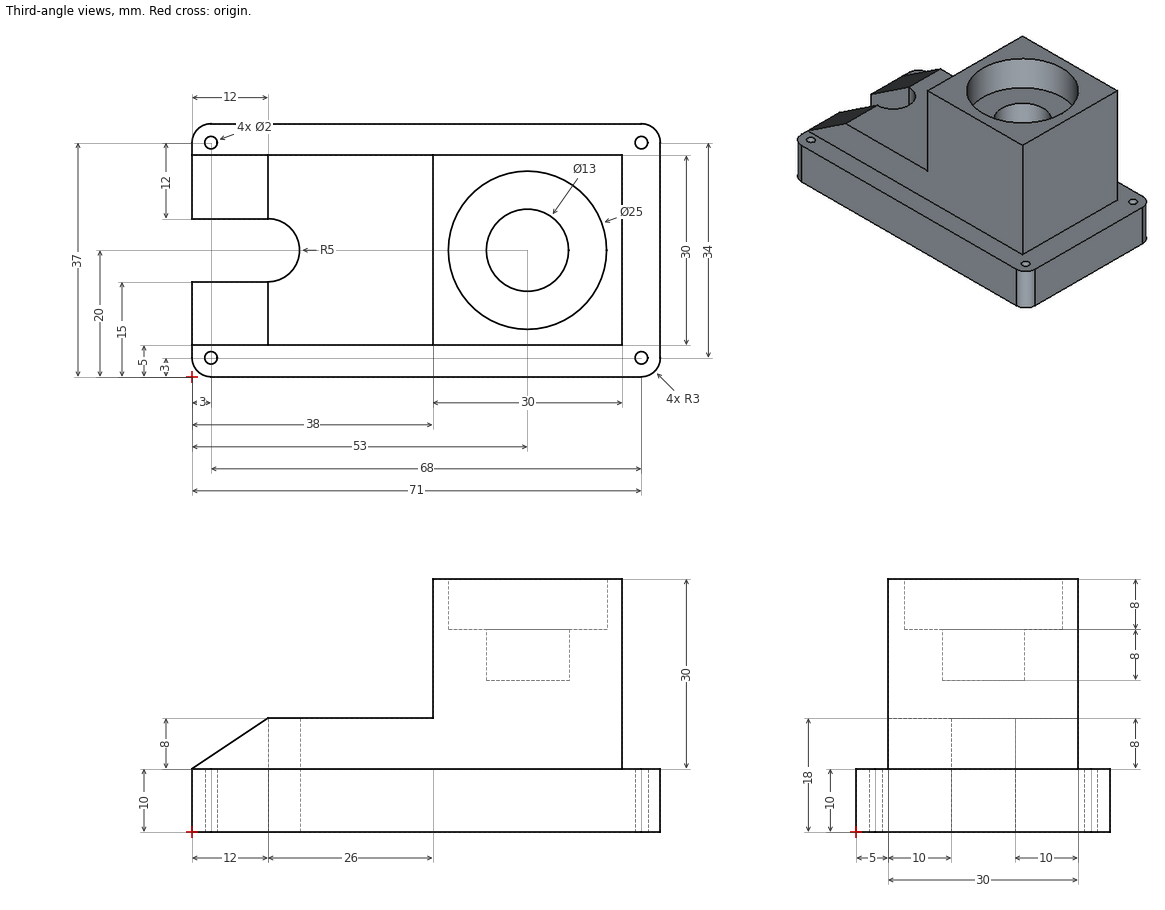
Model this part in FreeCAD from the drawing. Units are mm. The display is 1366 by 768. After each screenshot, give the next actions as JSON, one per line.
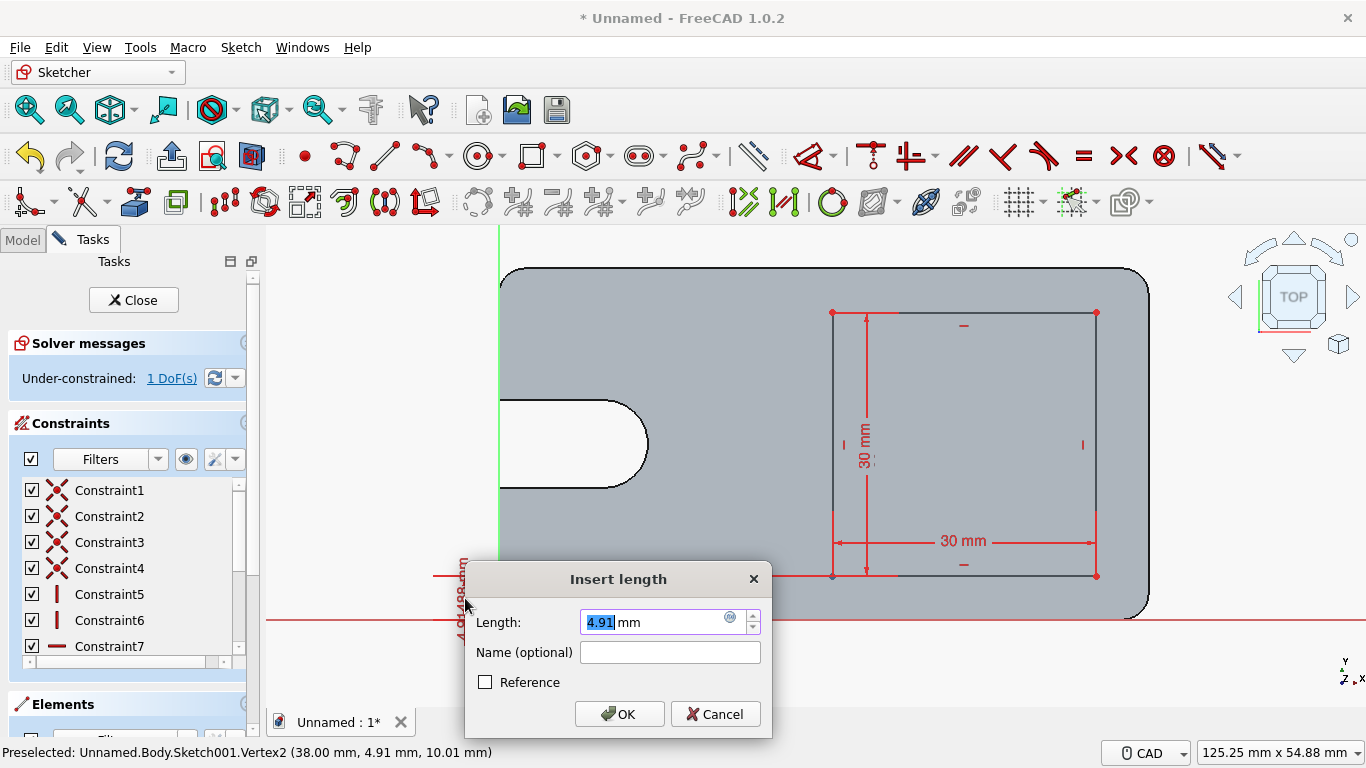
{"action": "type", "text": "5"}
{"action": "key", "text": "Return"}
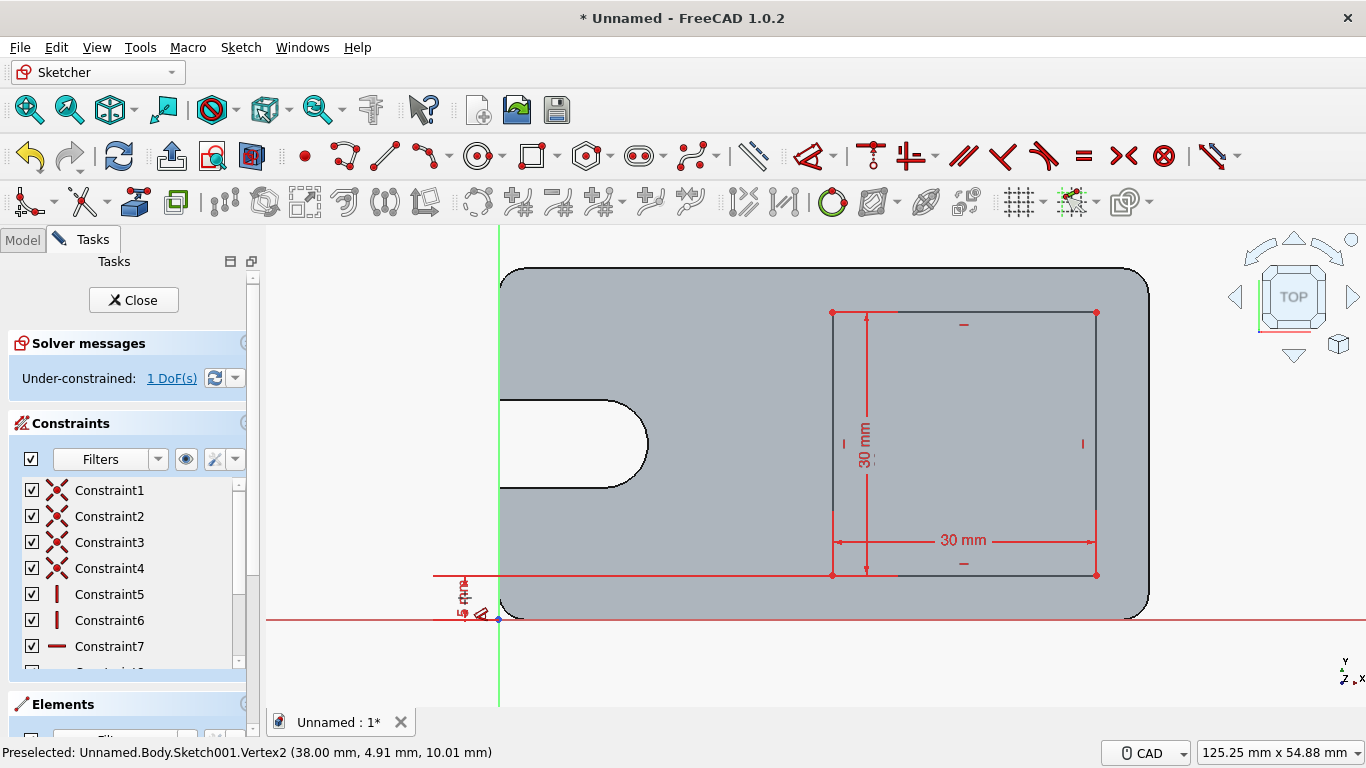
{"action": "left_click", "coordinate": [833, 312]}
{"action": "left_click", "coordinate": [666, 654]}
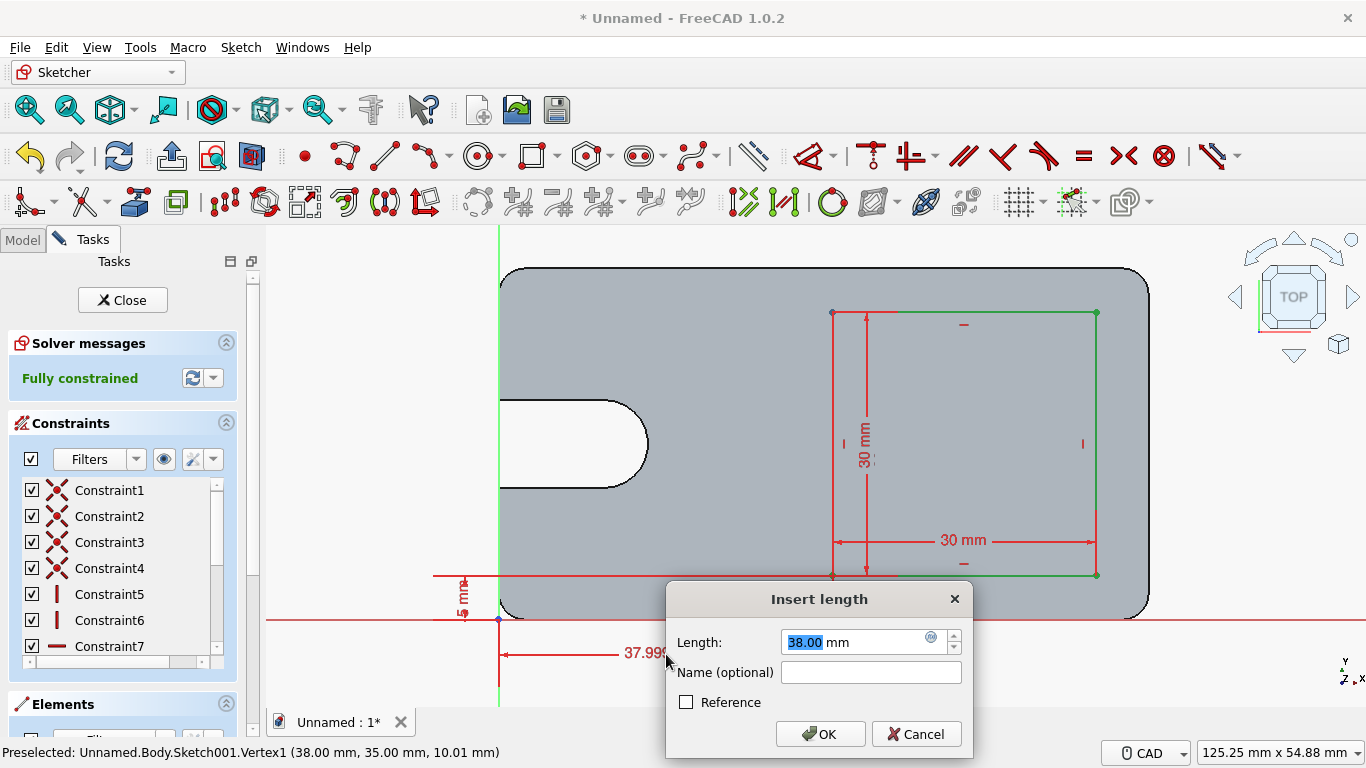
{"action": "type", "text": "38"}
{"action": "key", "text": "Return"}
{"action": "key", "text": "Escape"}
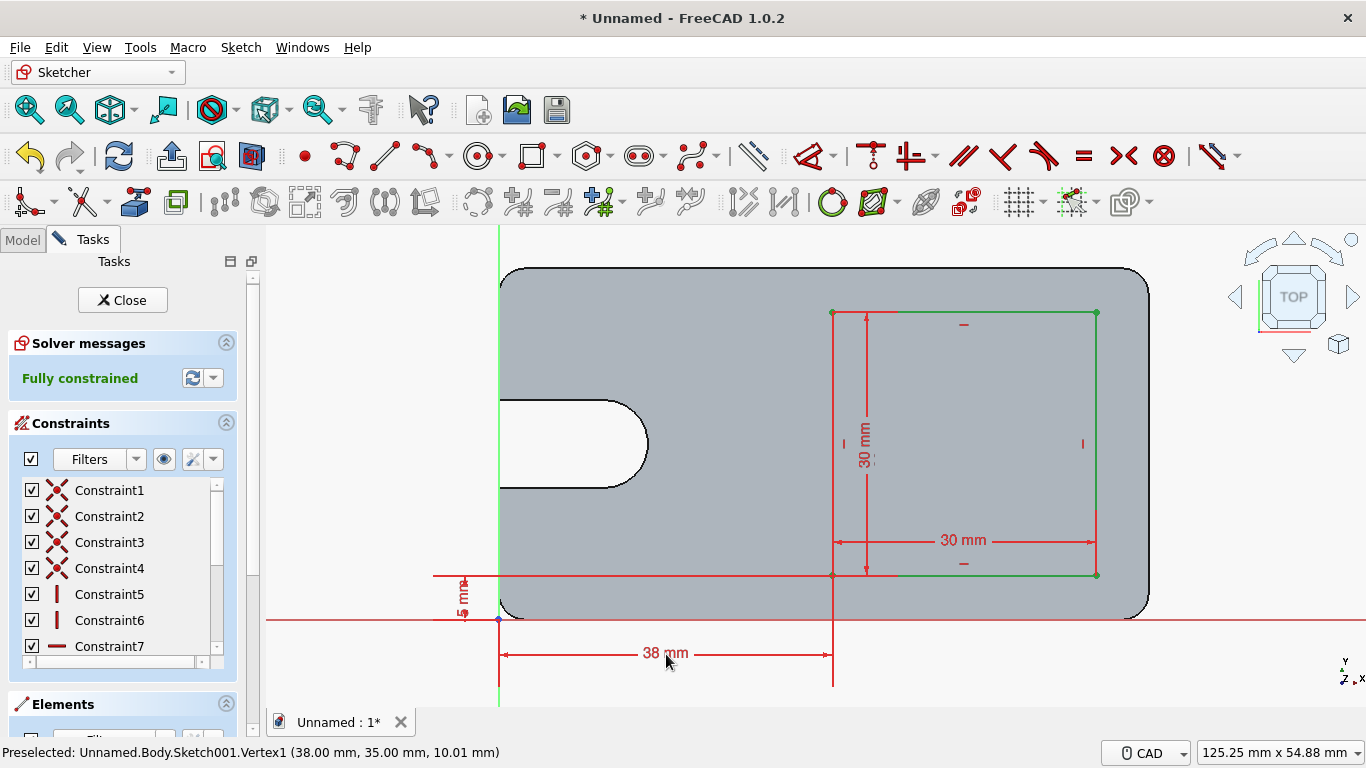
{"action": "left_click", "coordinate": [123, 300]}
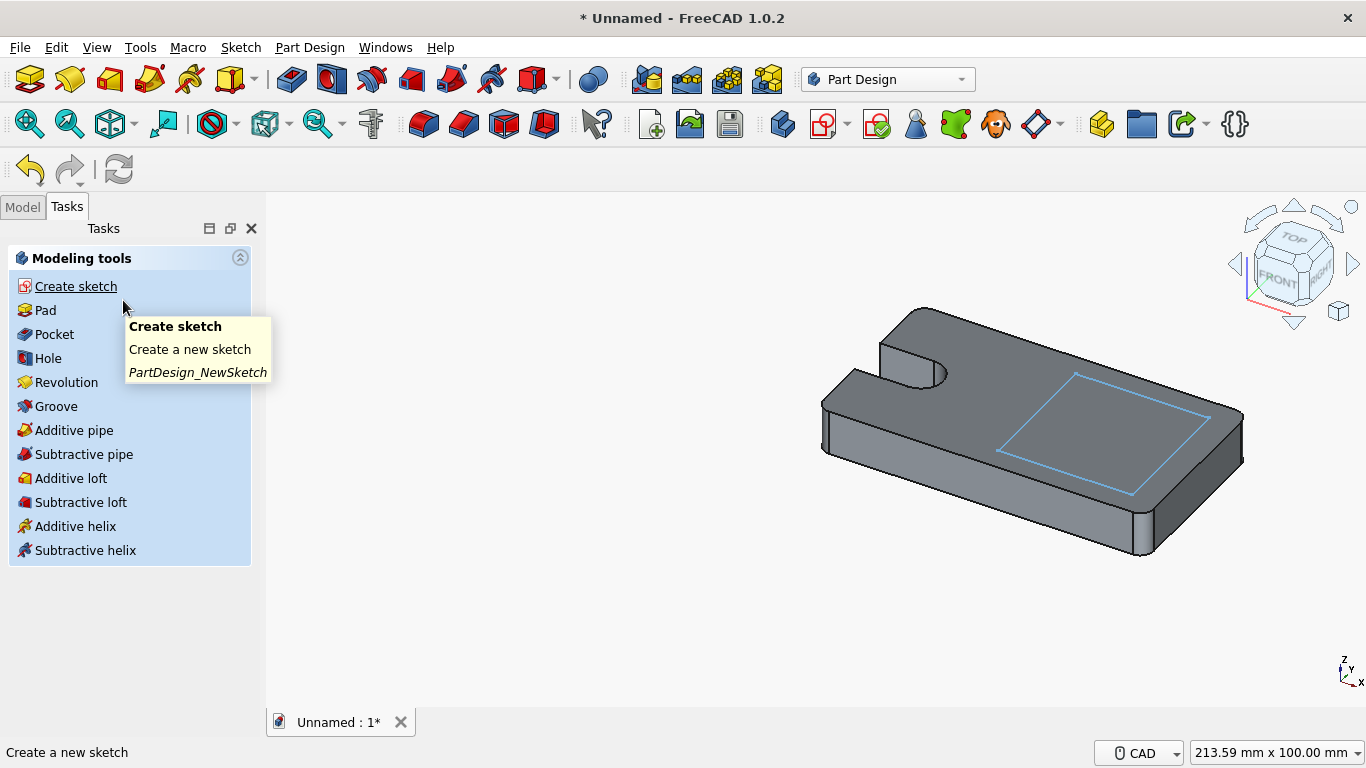
{"action": "left_click", "coordinate": [30, 80]}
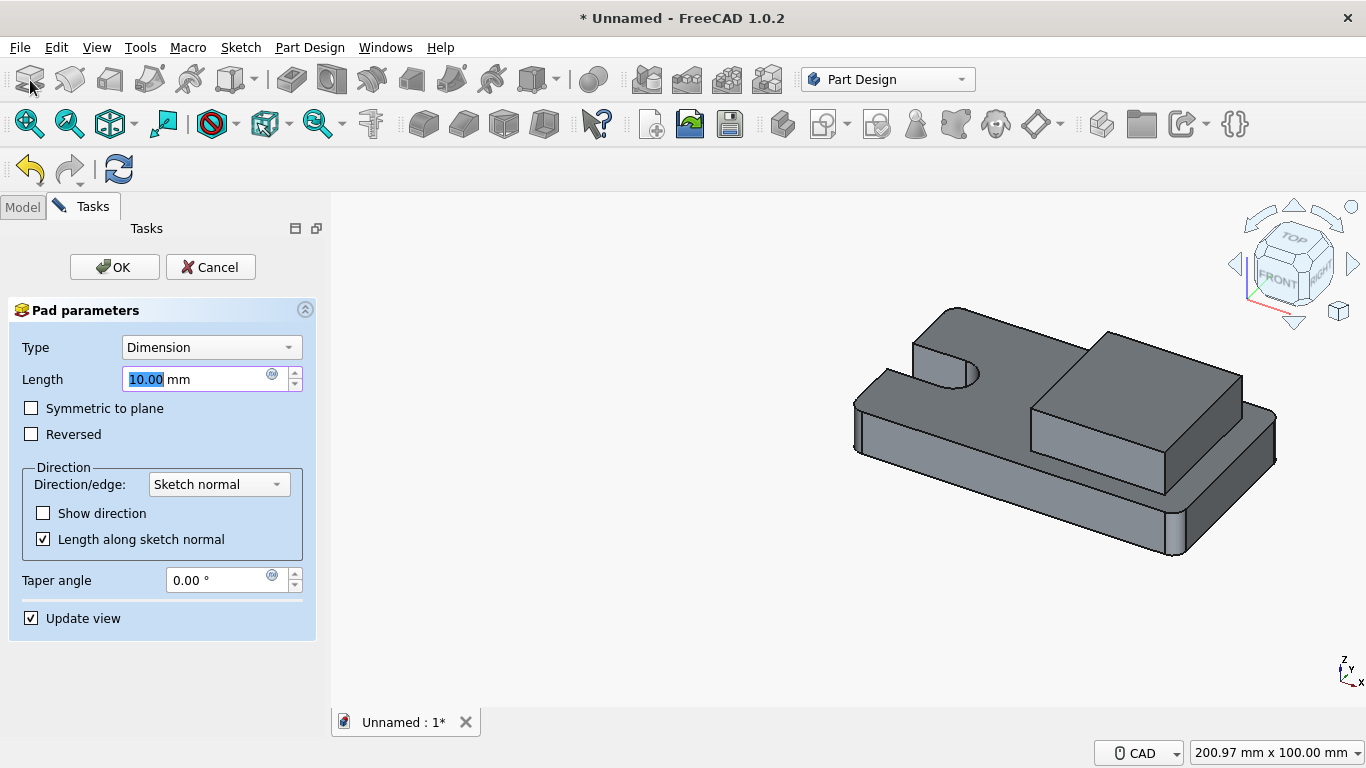
{"action": "type", "text": "30"}
{"action": "key", "text": "Tab"}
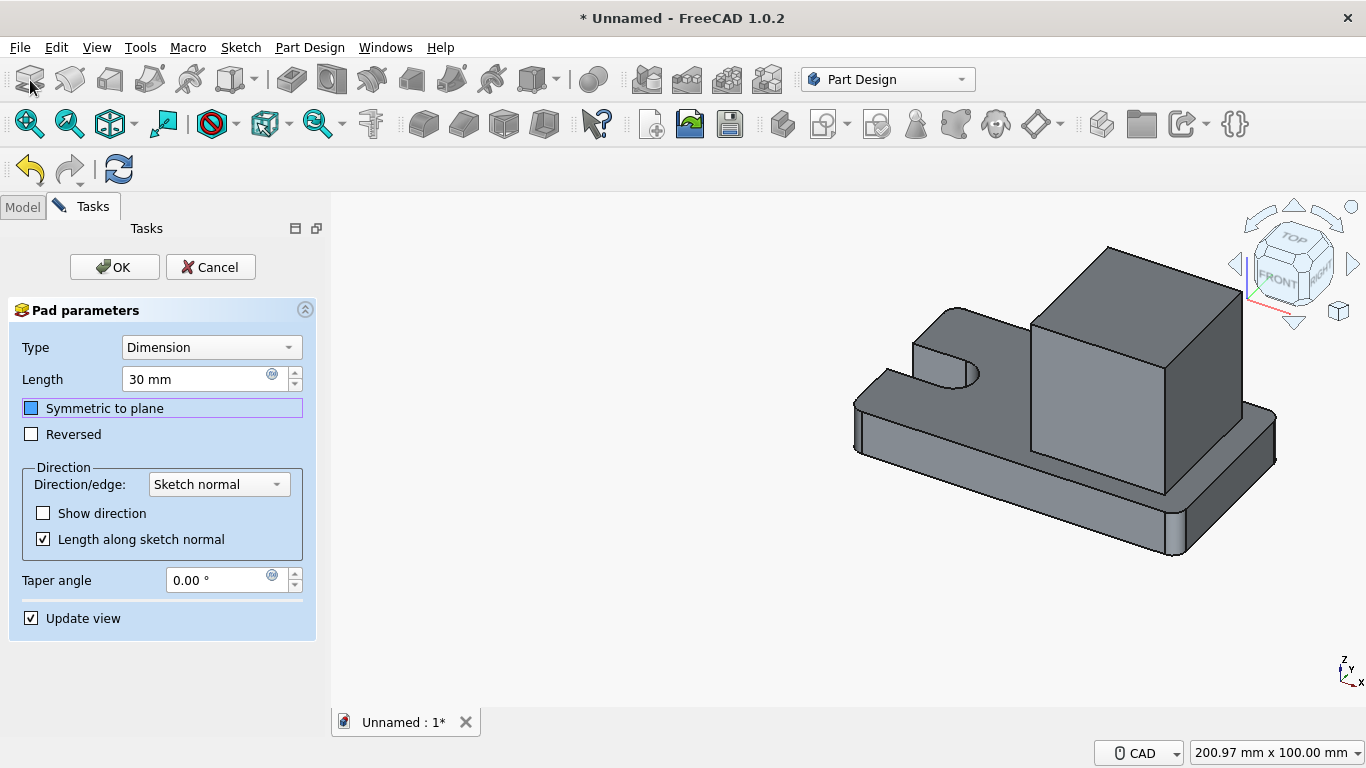
{"action": "left_click", "coordinate": [115, 267]}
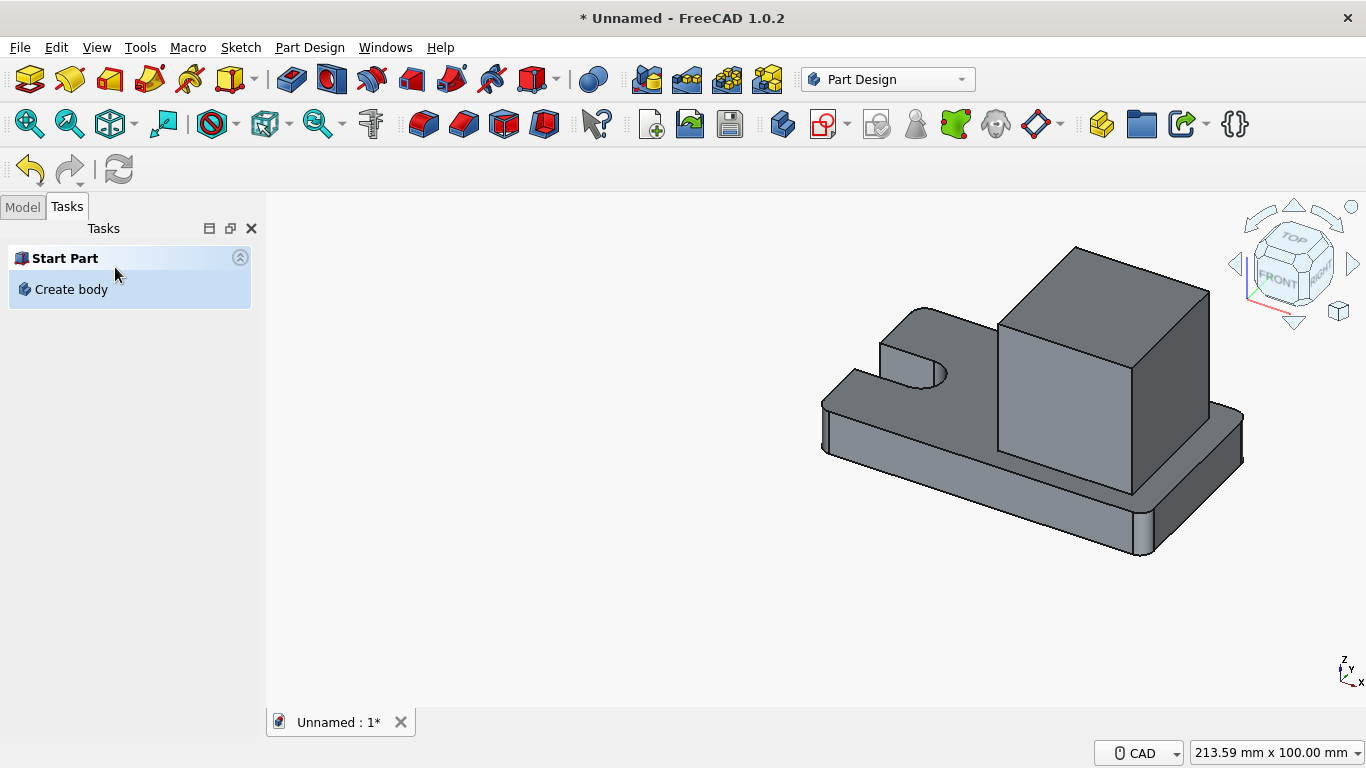
{"action": "key", "text": "v f"}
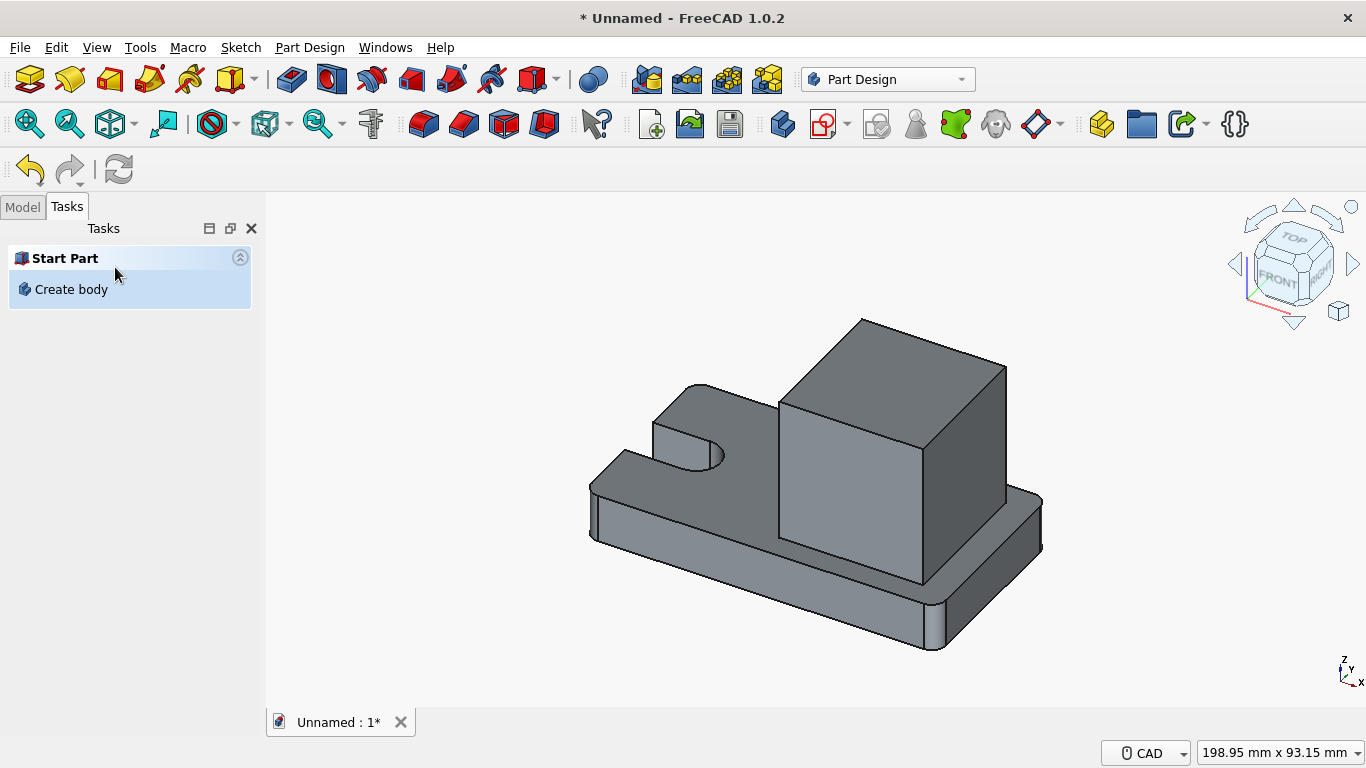
{"action": "key", "text": "6"}